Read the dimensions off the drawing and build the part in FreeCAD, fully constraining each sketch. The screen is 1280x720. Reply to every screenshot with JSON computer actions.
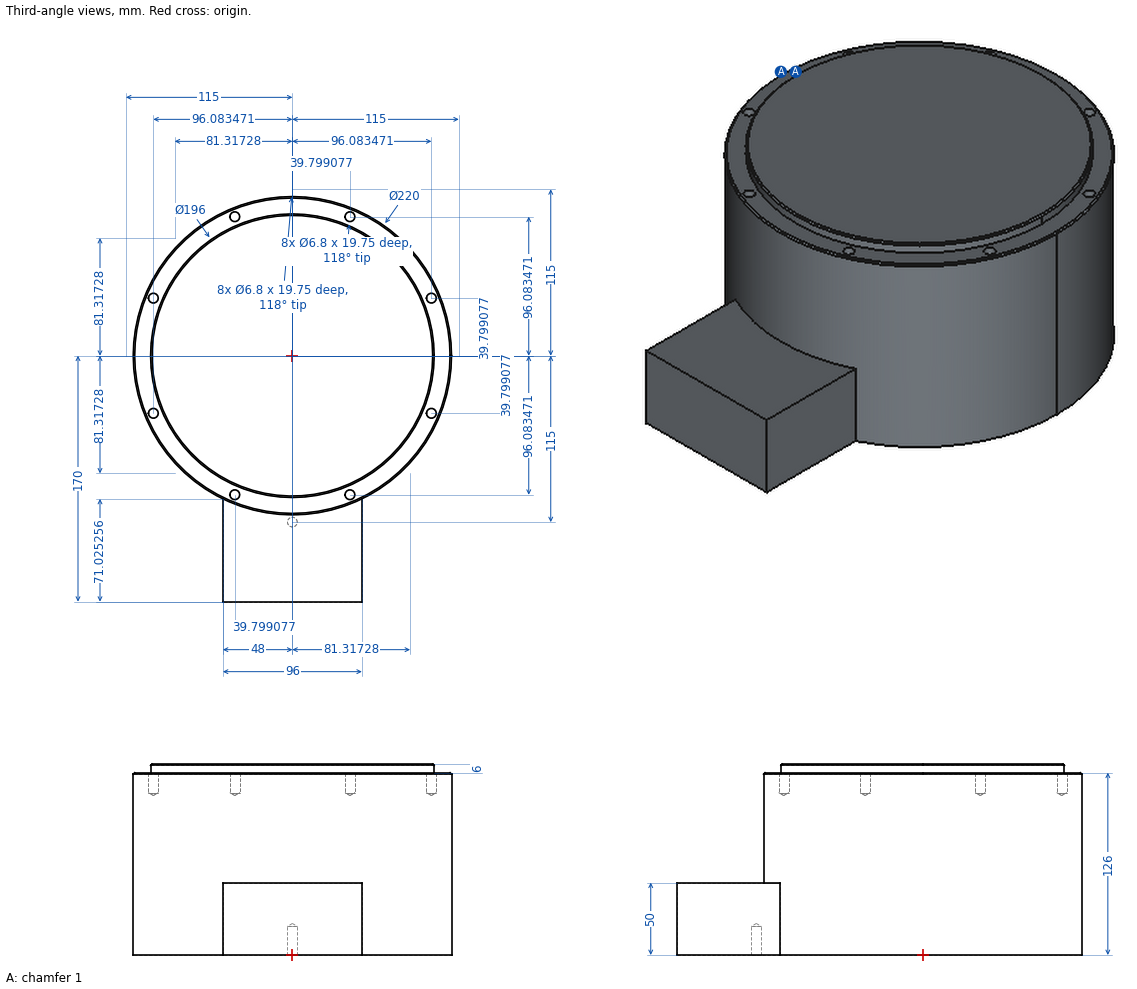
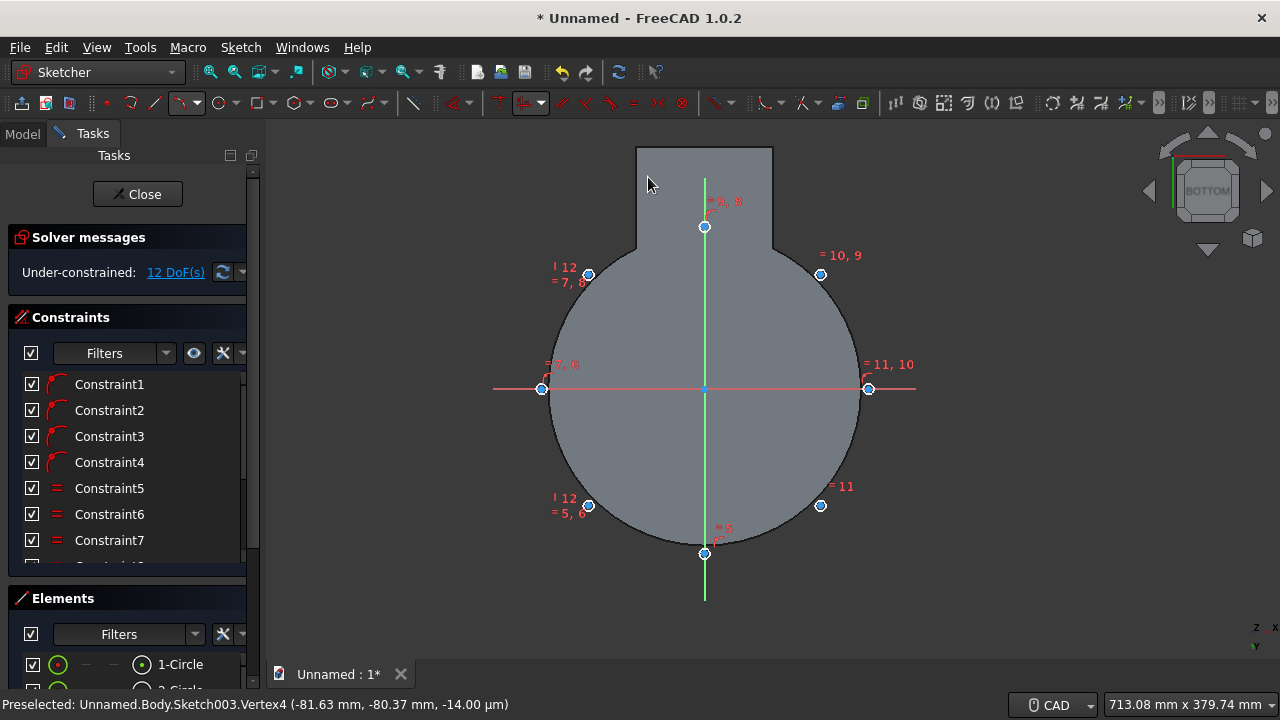
{"action": "left_click", "coordinate": [589, 275]}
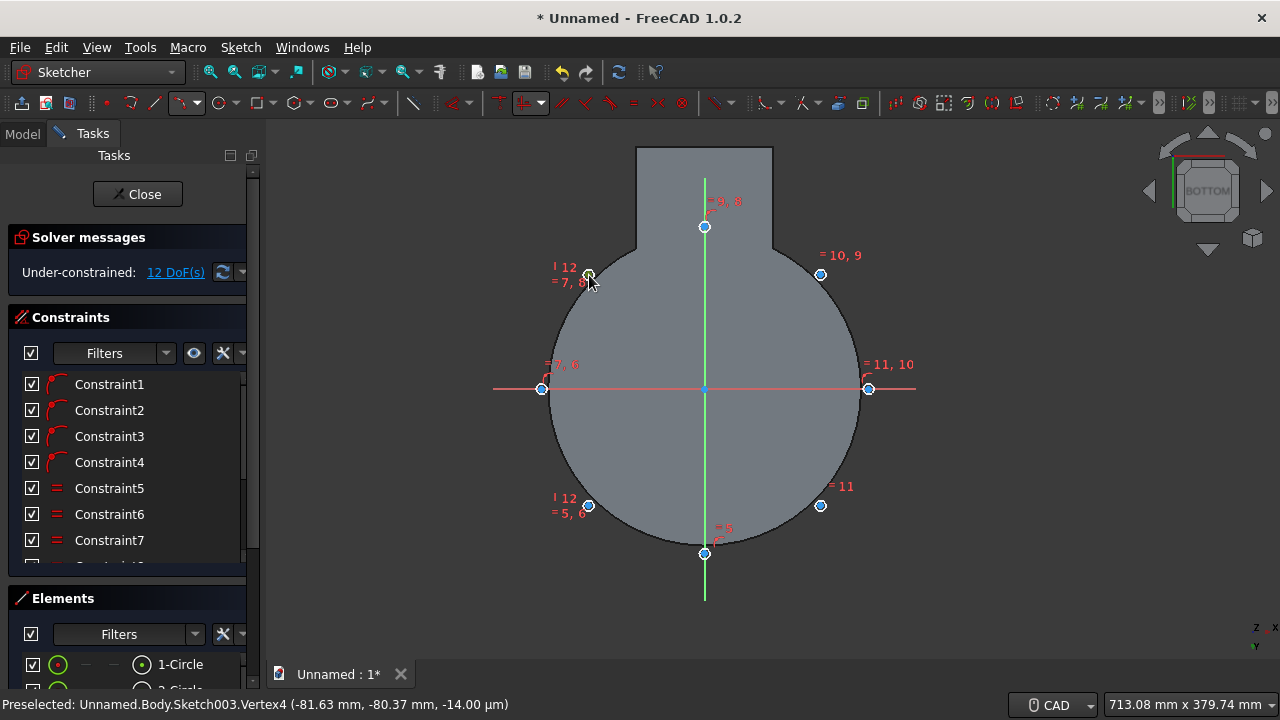
{"action": "left_click", "coordinate": [821, 275]}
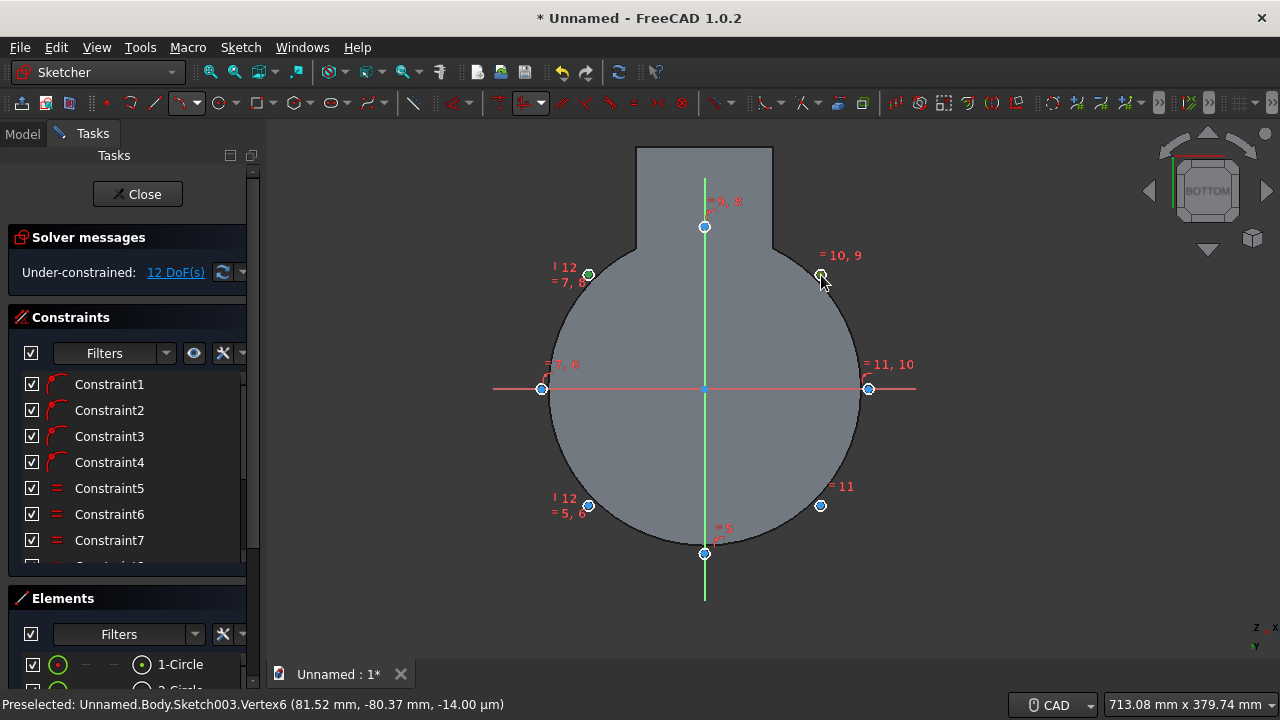
{"action": "left_click", "coordinate": [544, 104]}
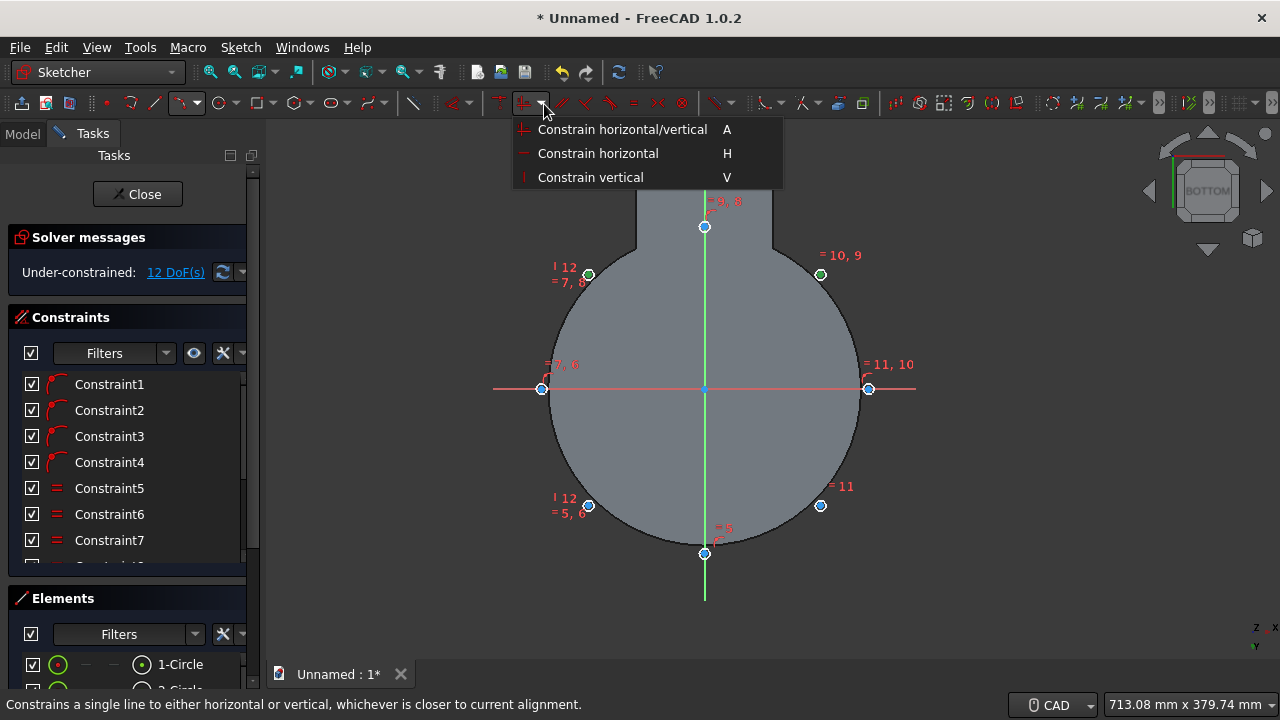
{"action": "left_click", "coordinate": [648, 153]}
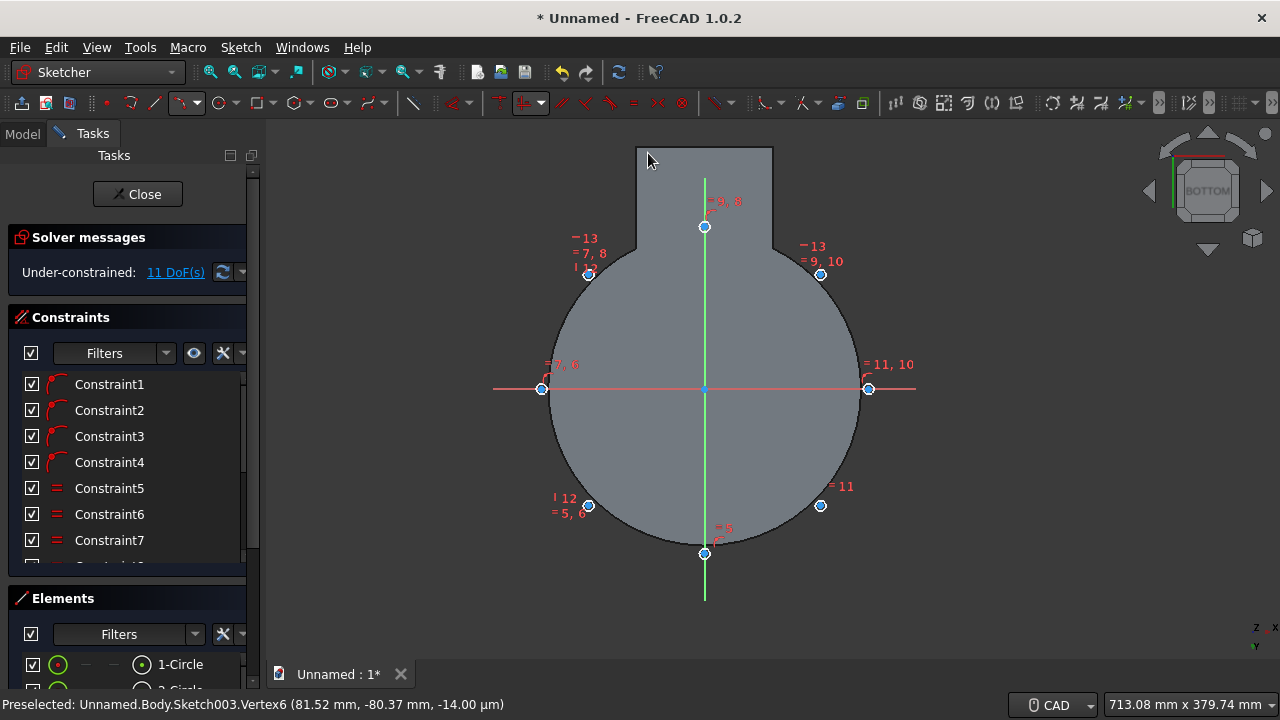
{"action": "left_click", "coordinate": [821, 275]}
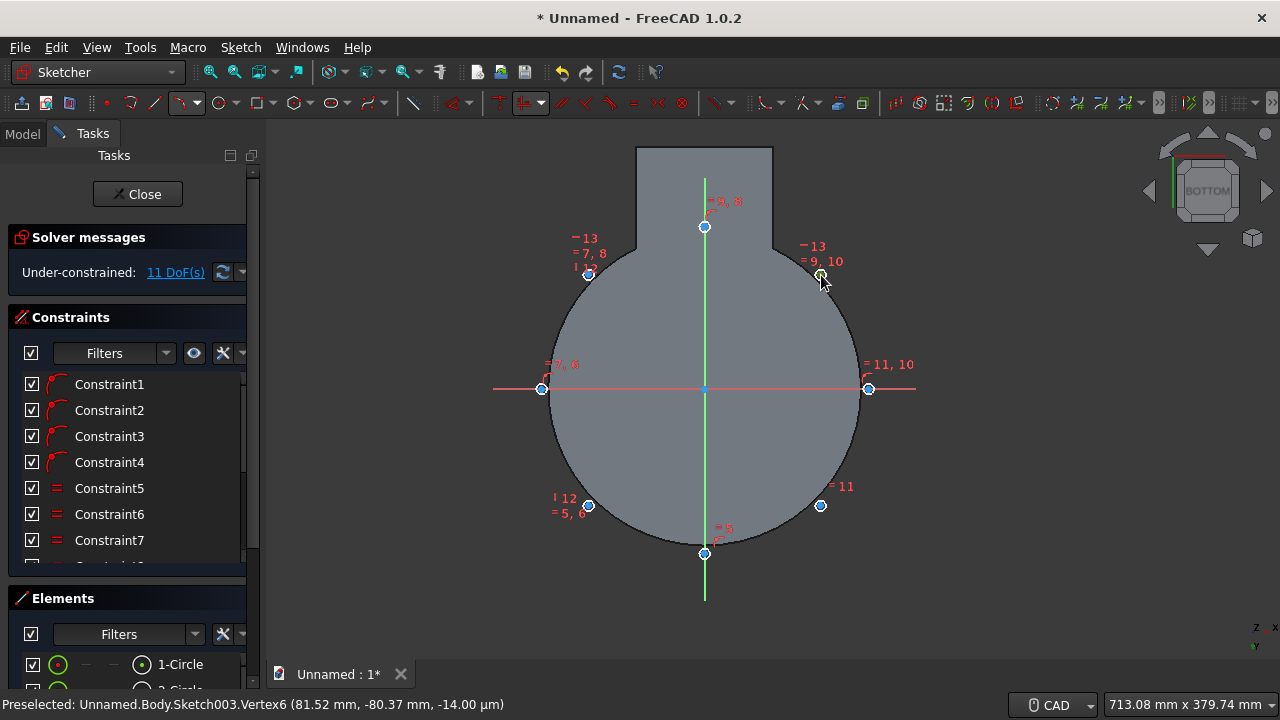
{"action": "left_click", "coordinate": [821, 506]}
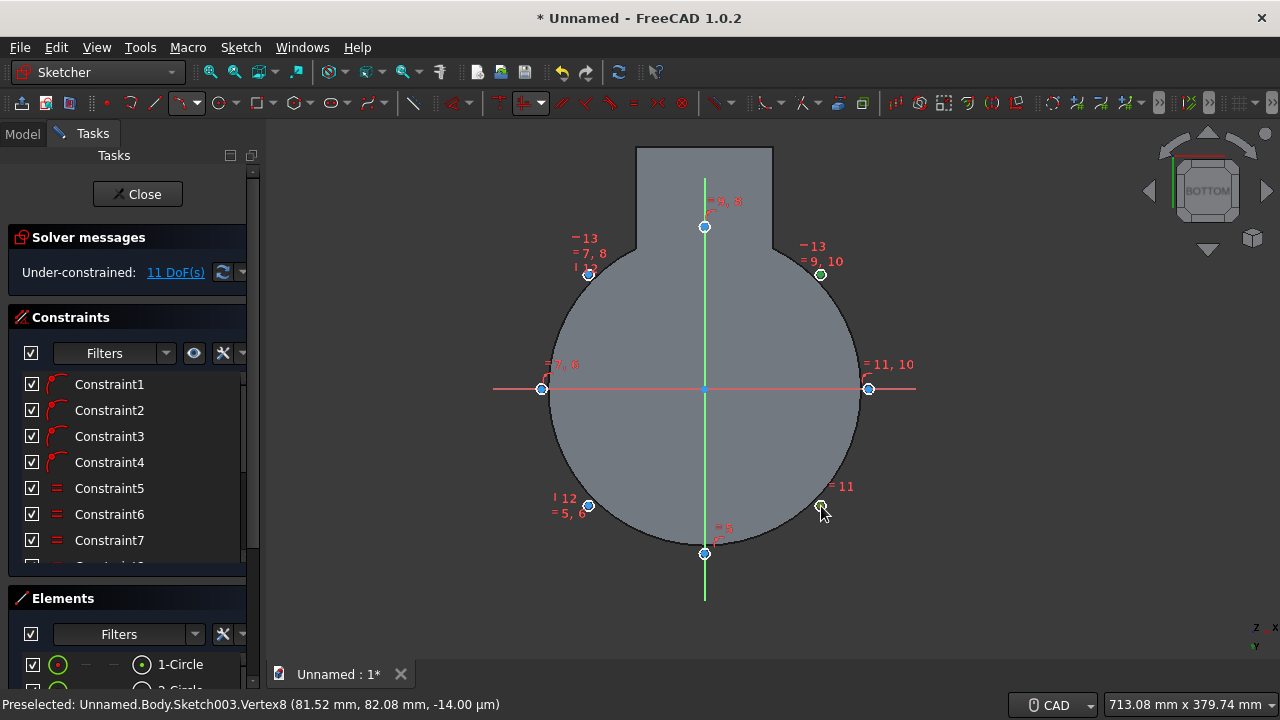
{"action": "left_click", "coordinate": [544, 104]}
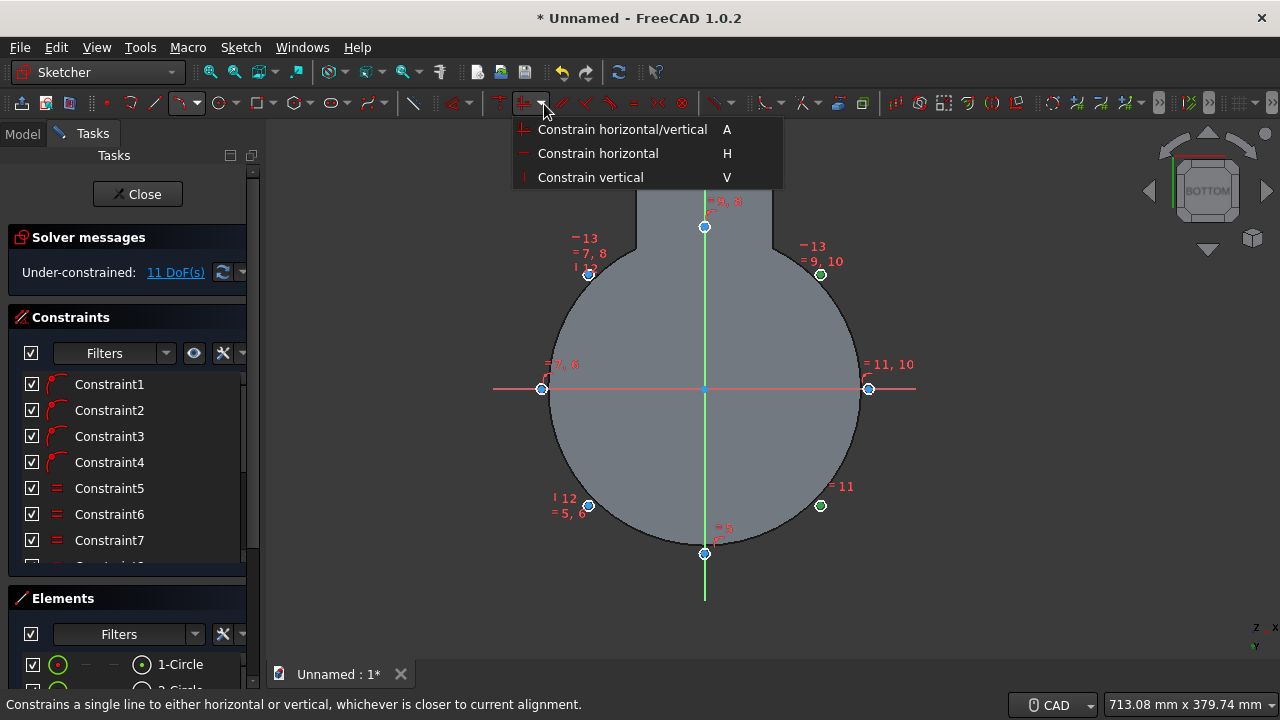
{"action": "left_click", "coordinate": [648, 177]}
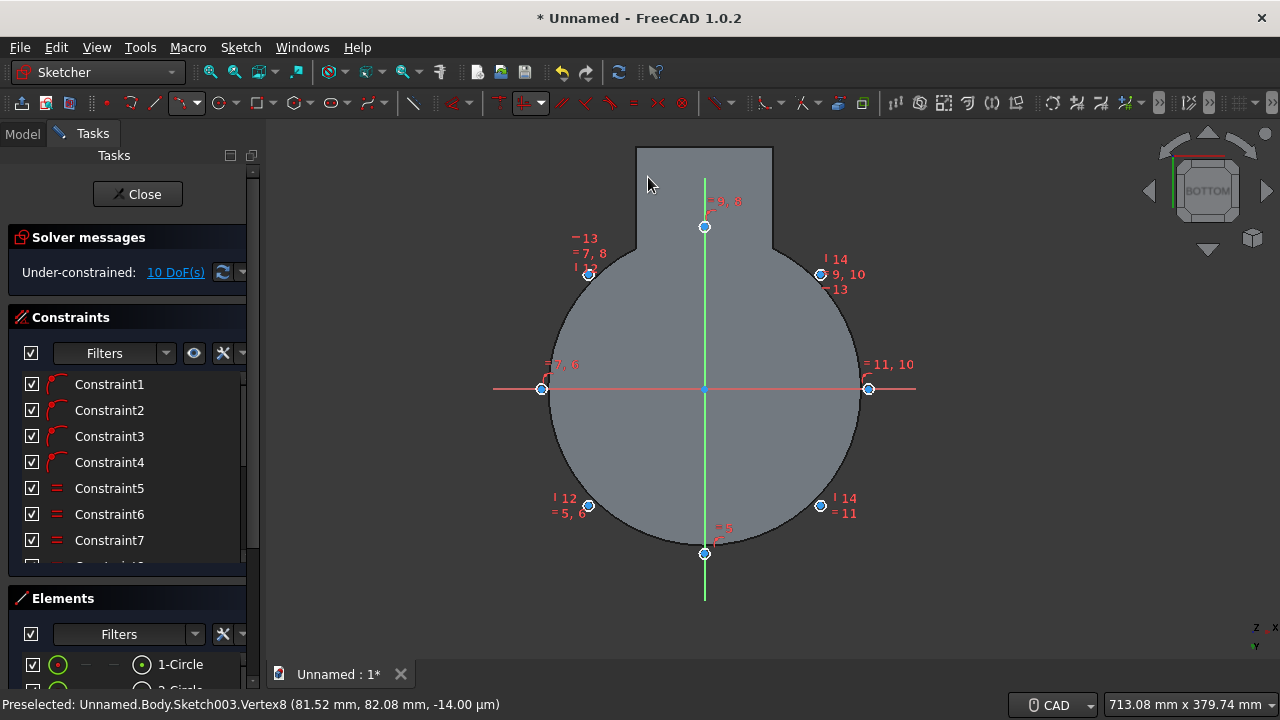
{"action": "left_click", "coordinate": [589, 506]}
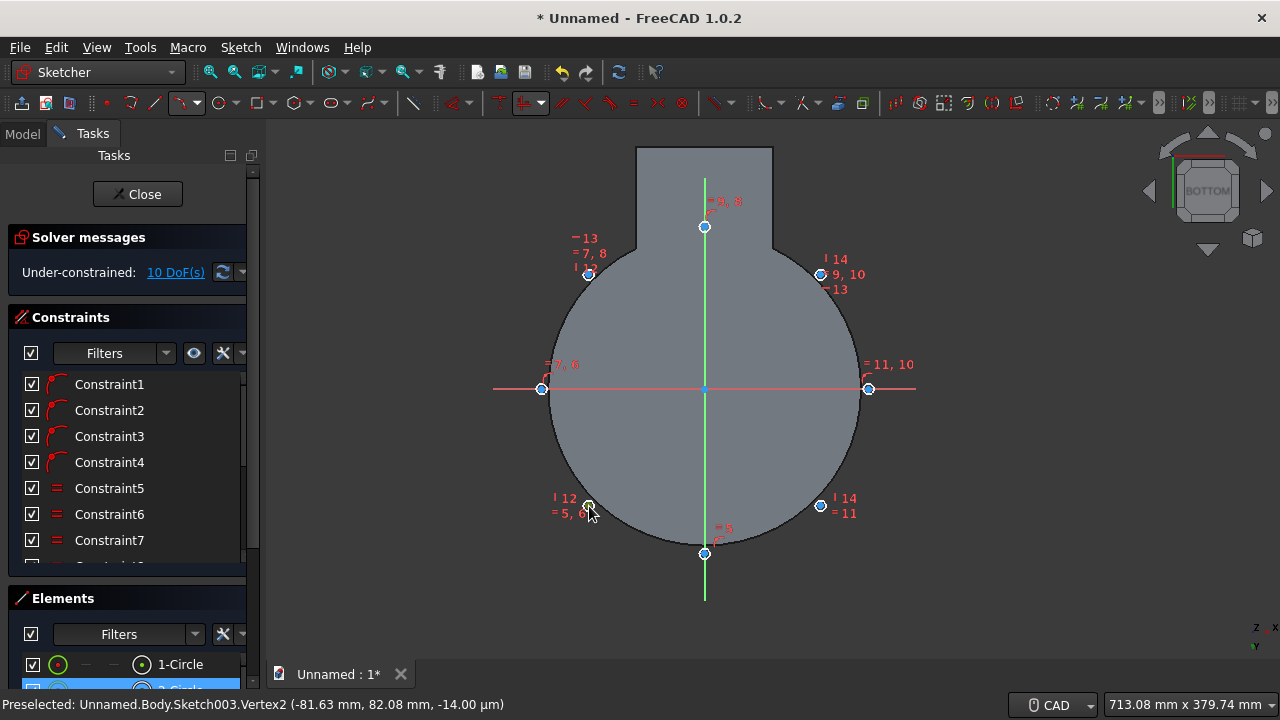
{"action": "left_click", "coordinate": [821, 506]}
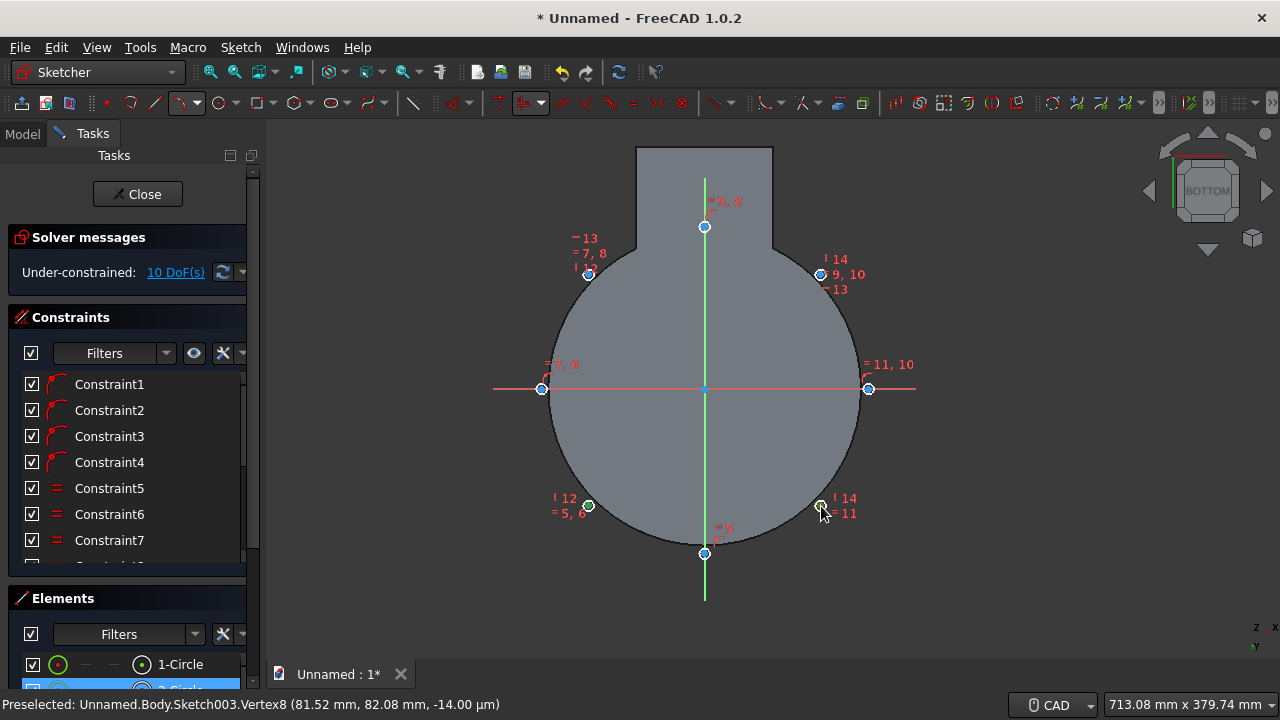
{"action": "left_click", "coordinate": [544, 104]}